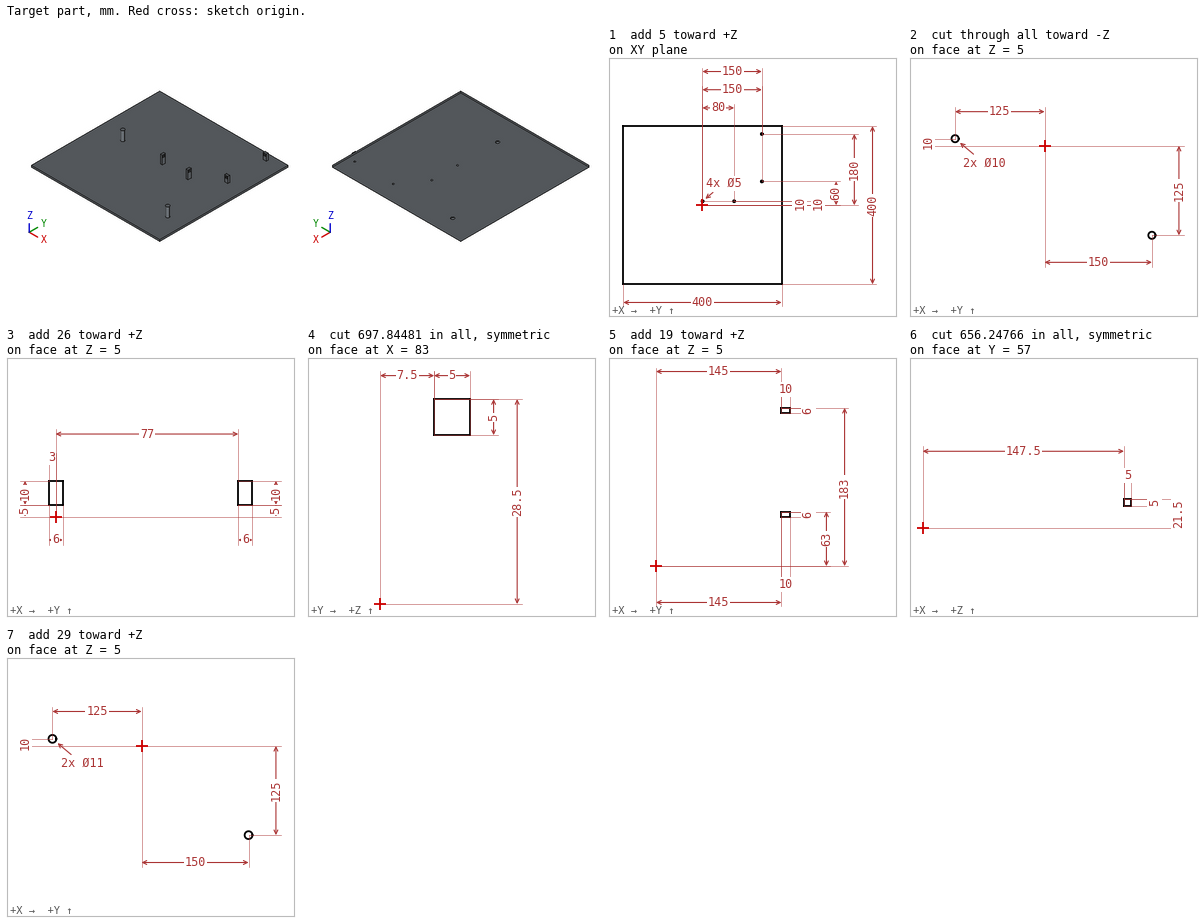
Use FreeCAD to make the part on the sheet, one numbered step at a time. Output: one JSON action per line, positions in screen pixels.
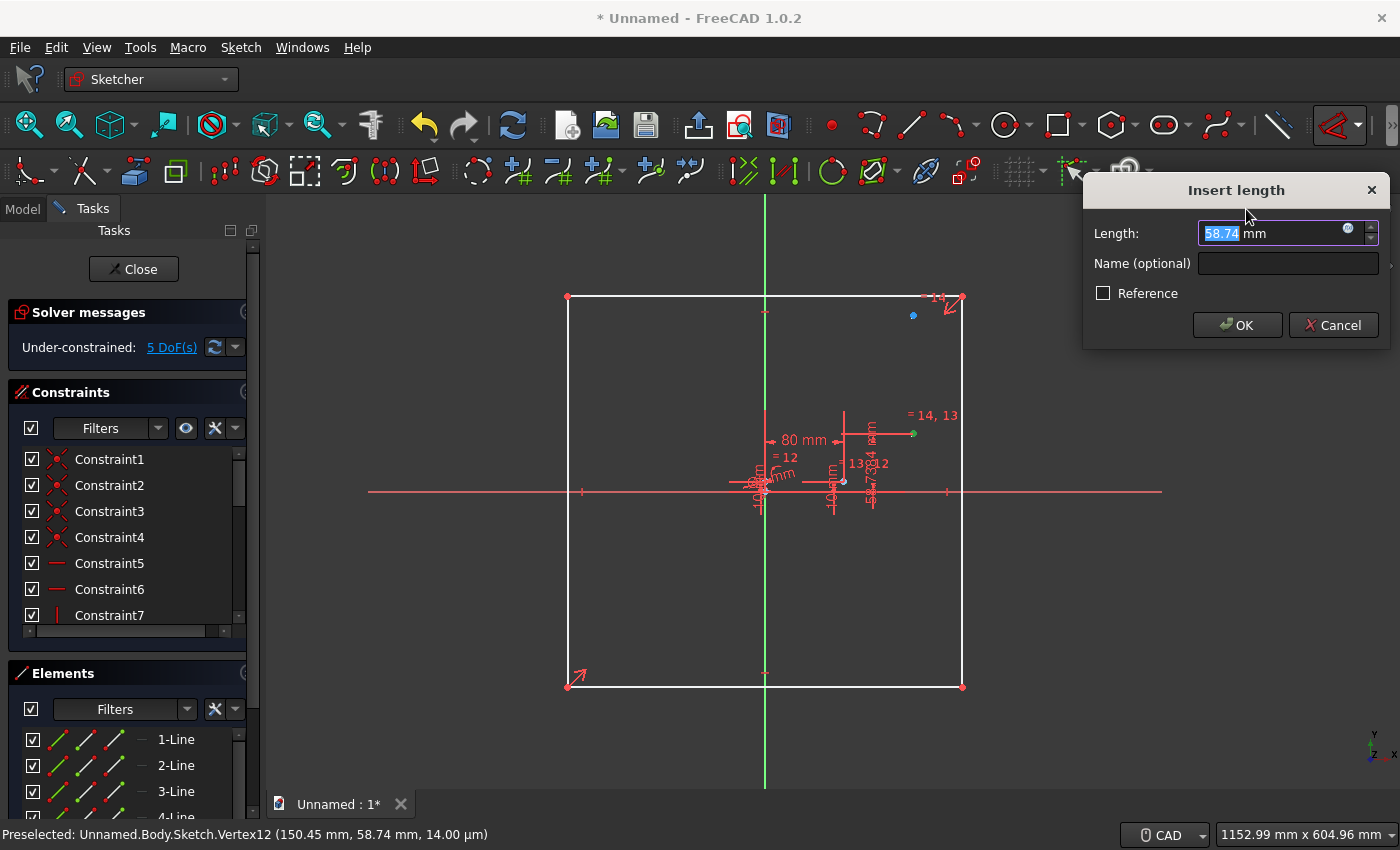
{"action": "type", "text": "60"}
{"action": "key", "text": "Return"}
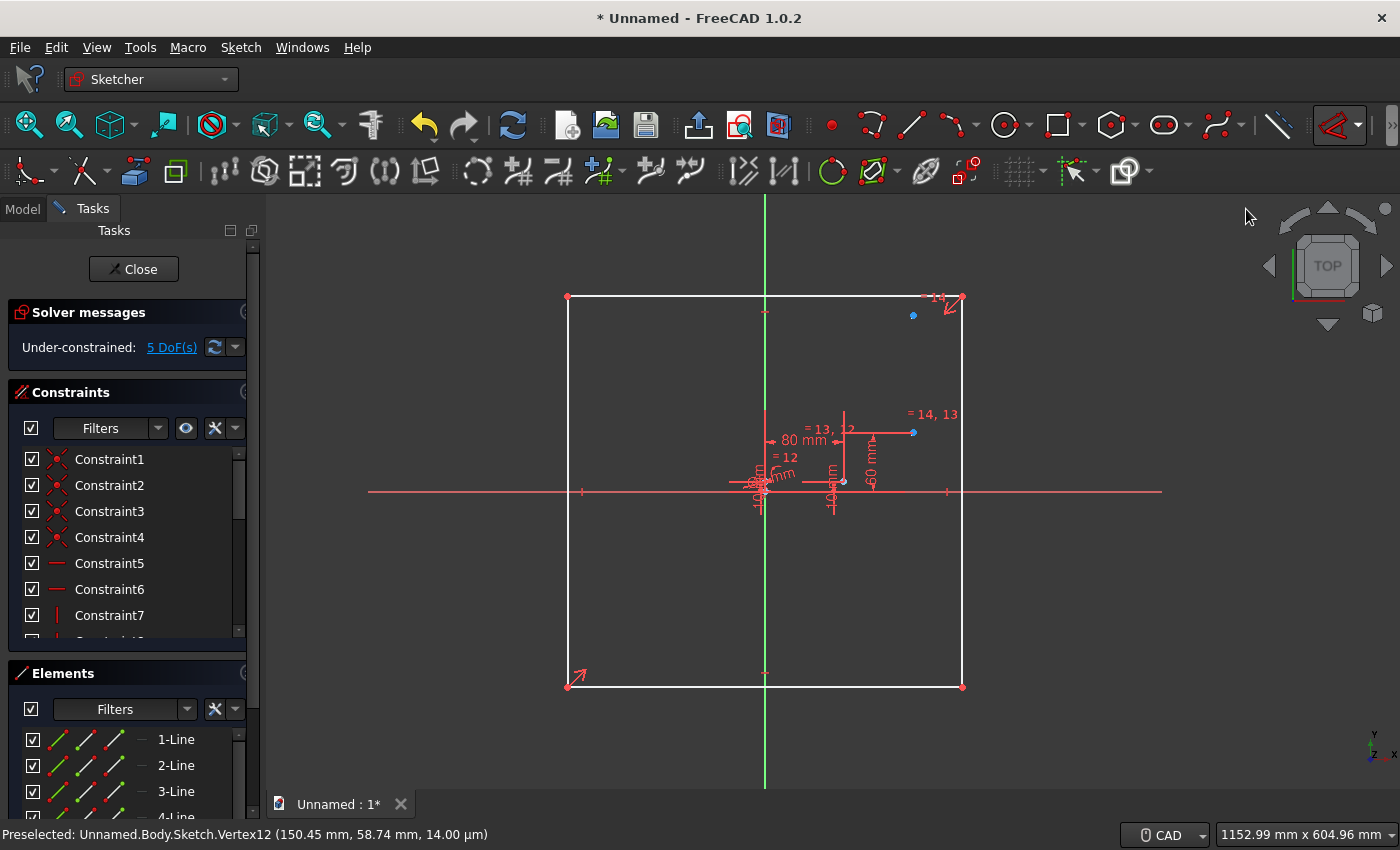
{"action": "left_click", "coordinate": [686, 687]}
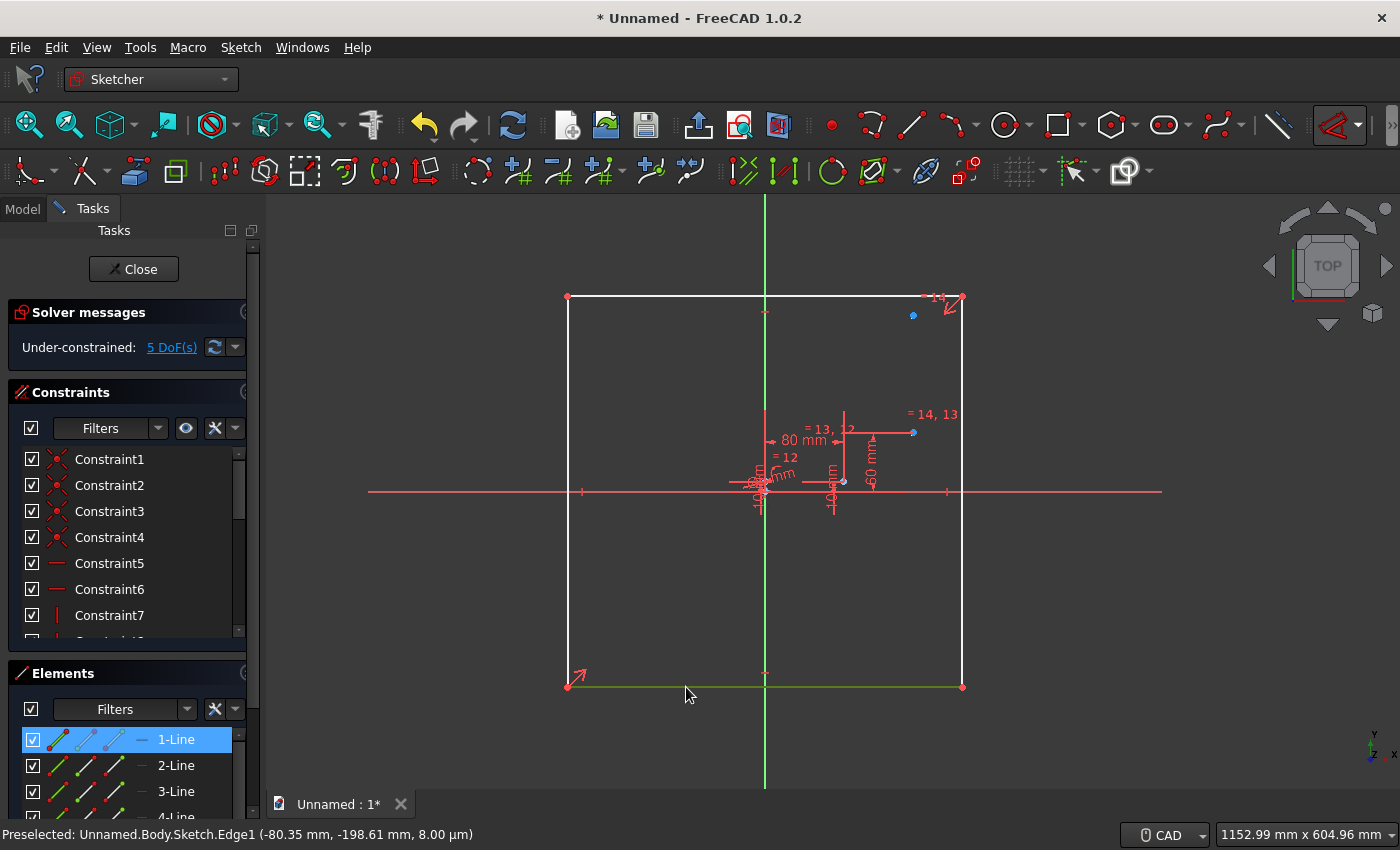
{"action": "key", "text": "l"}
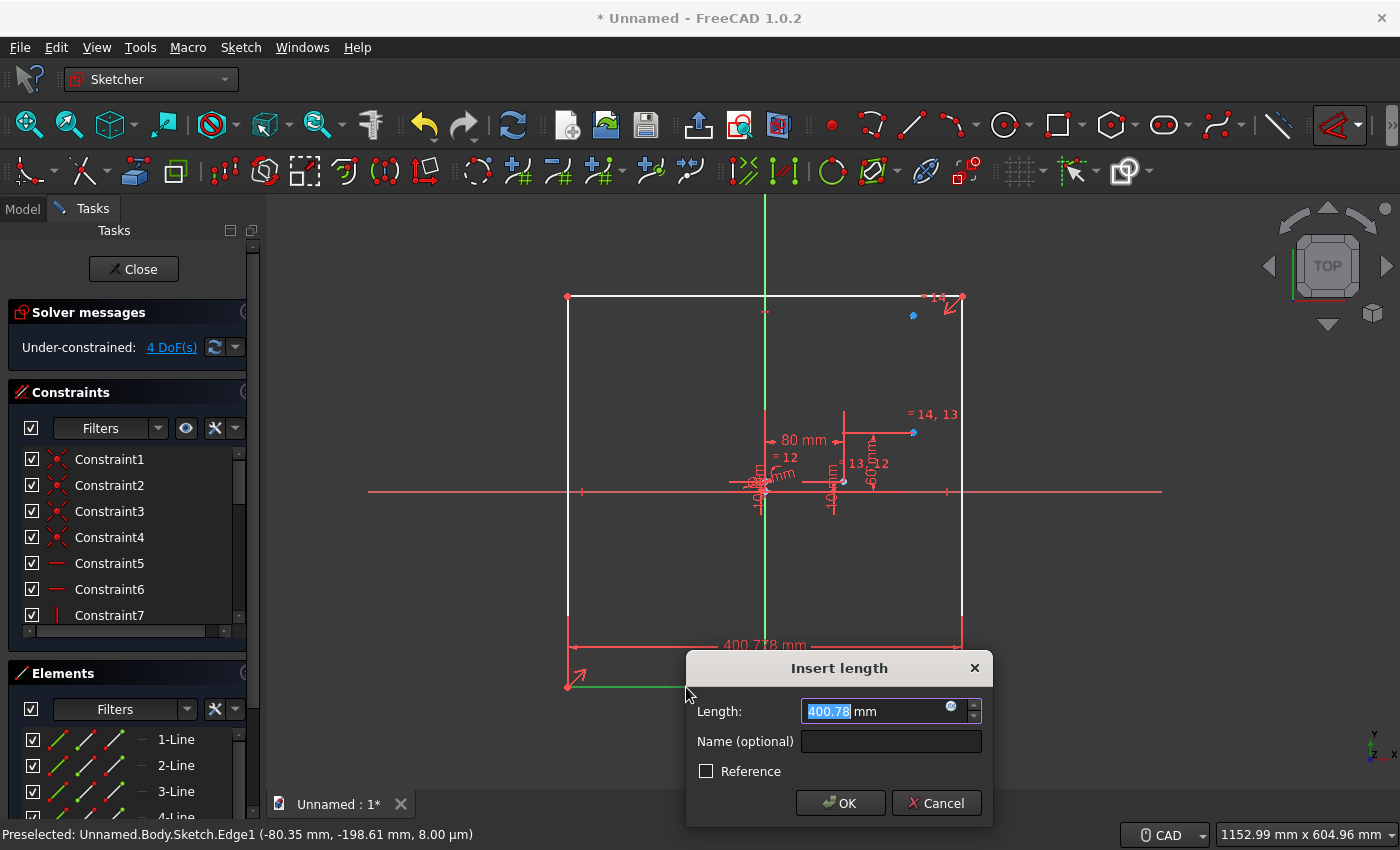
{"action": "type", "text": "400"}
{"action": "key", "text": "Return"}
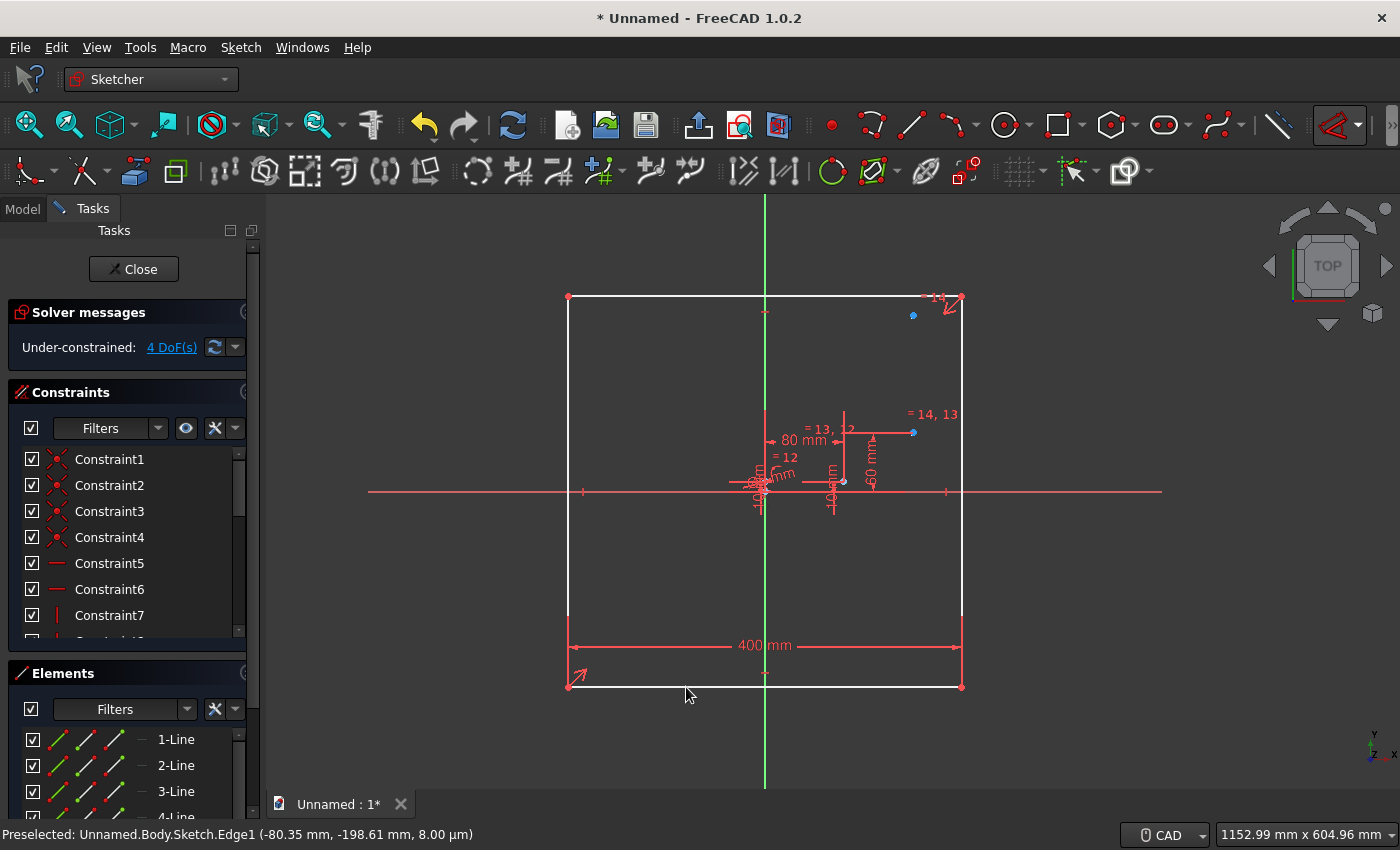
{"action": "left_click", "coordinate": [962, 570]}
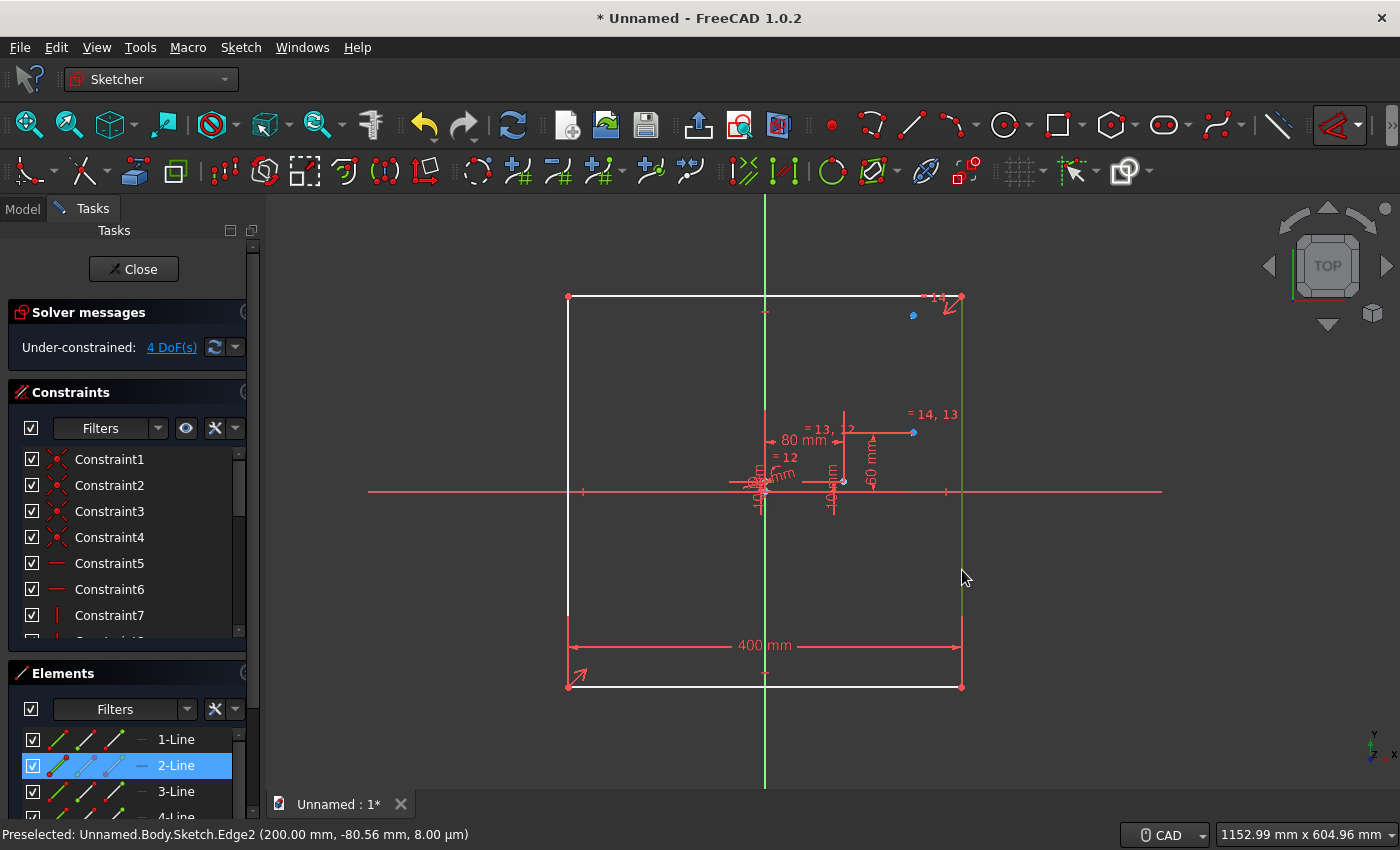
{"action": "key", "text": "i"}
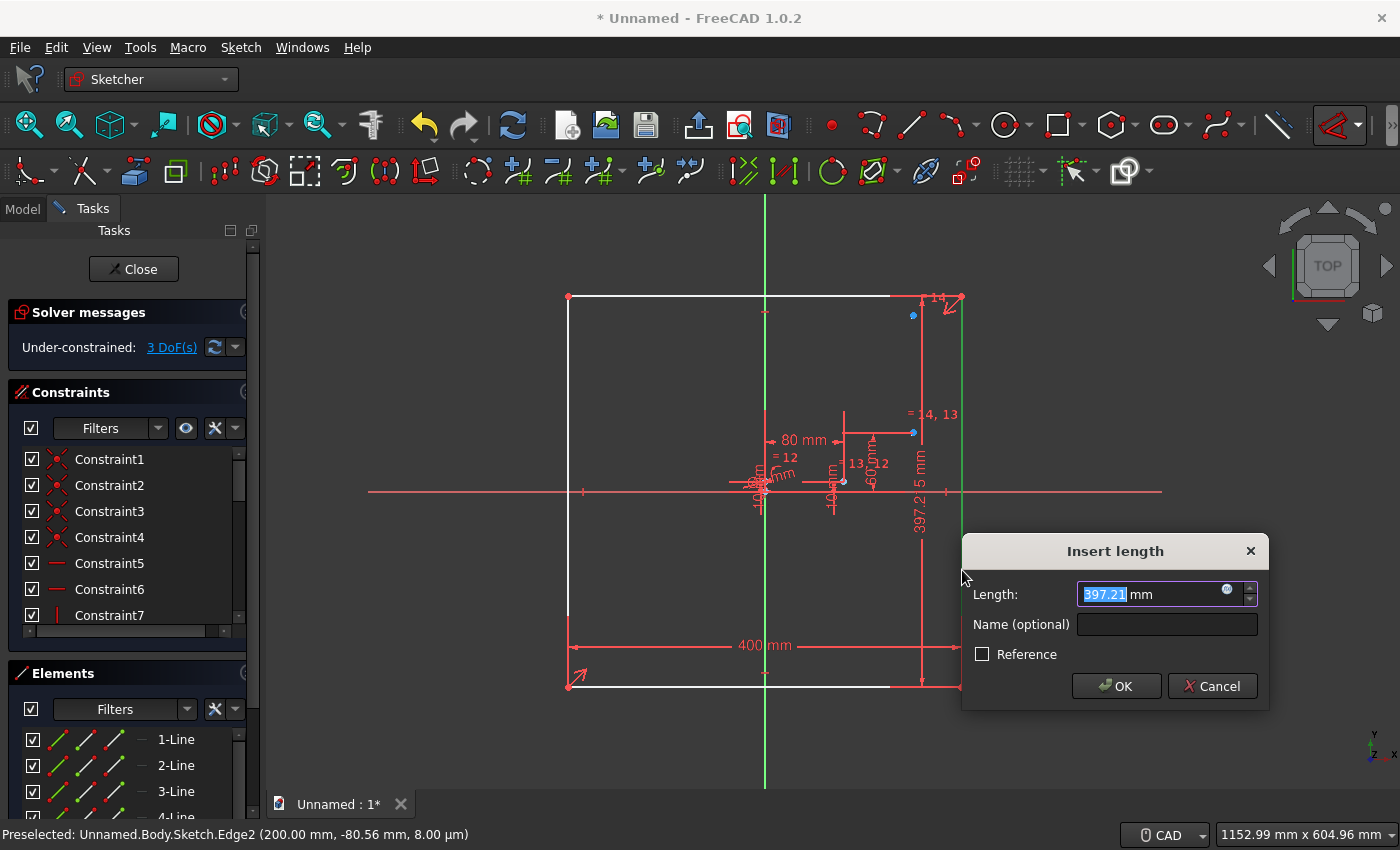
{"action": "type", "text": "400"}
{"action": "key", "text": "Return"}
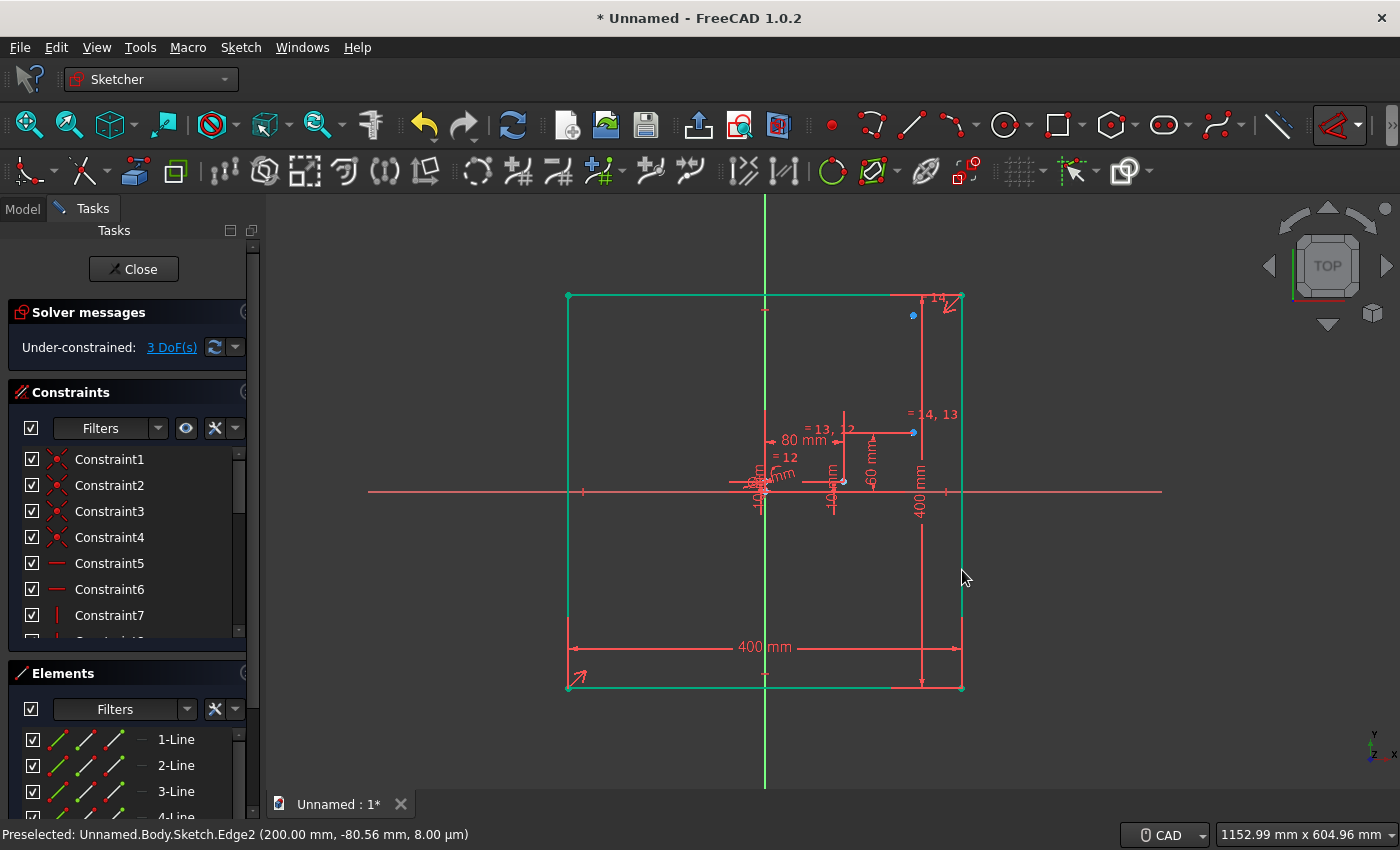
{"action": "left_click", "coordinate": [913, 433]}